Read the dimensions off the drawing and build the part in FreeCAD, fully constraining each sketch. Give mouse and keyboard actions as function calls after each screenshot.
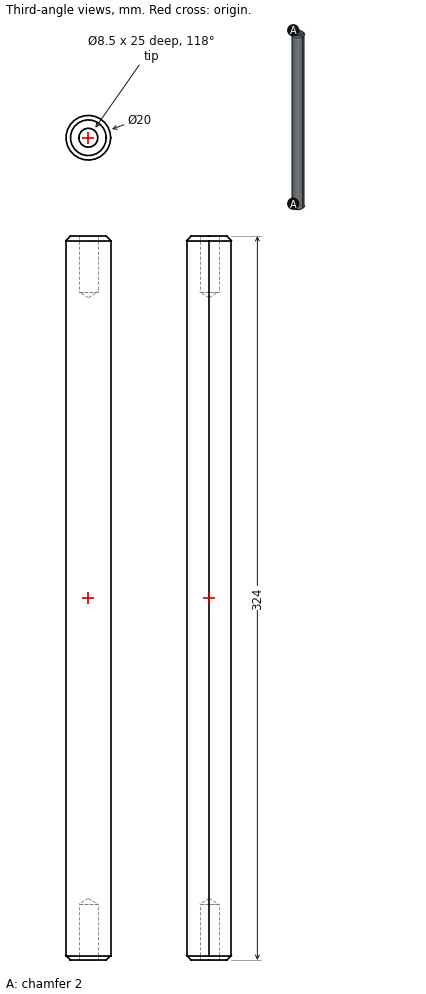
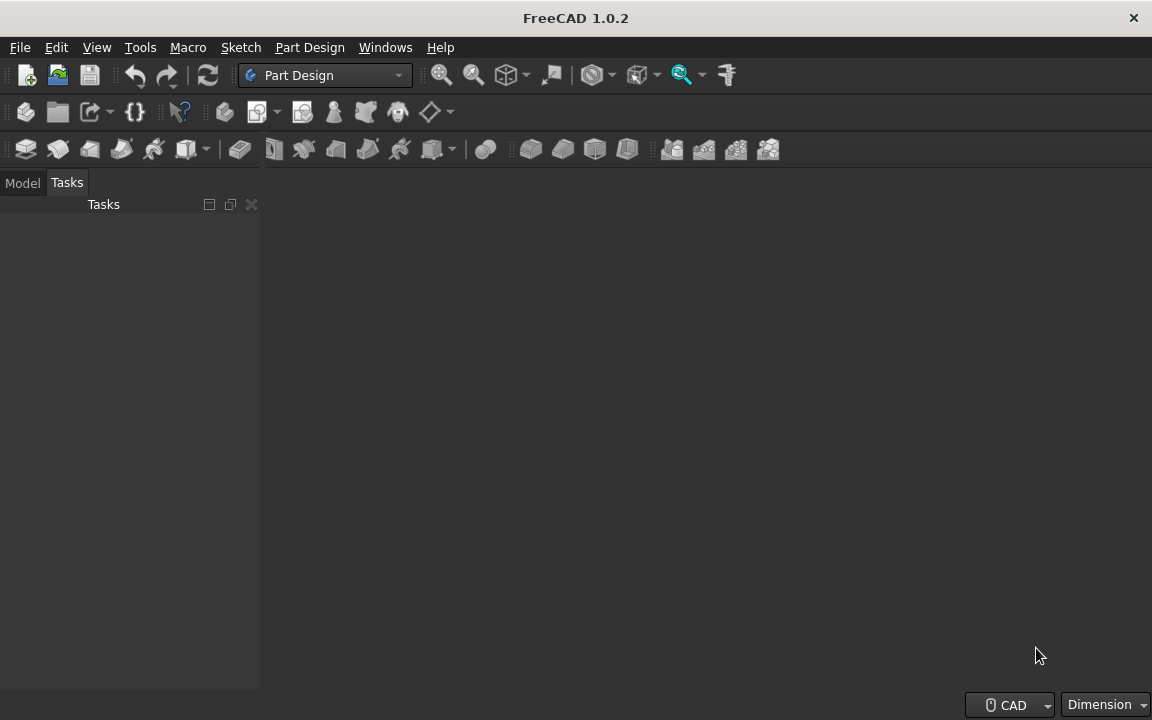
click(26, 76)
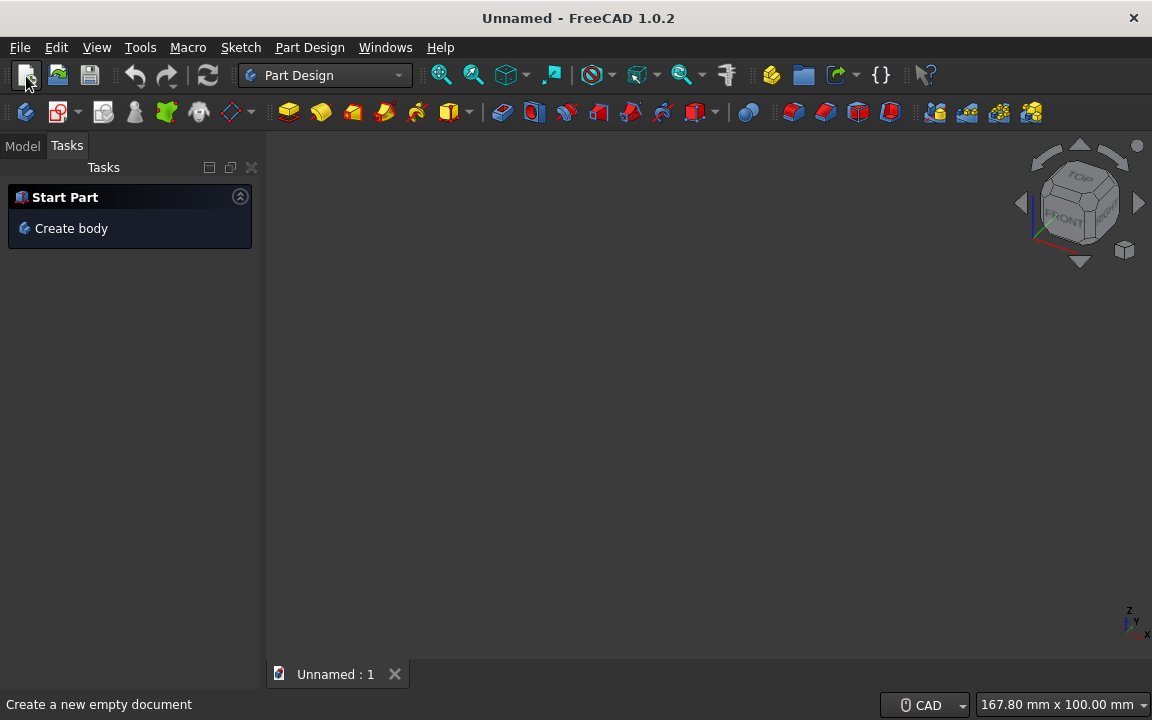
click(58, 112)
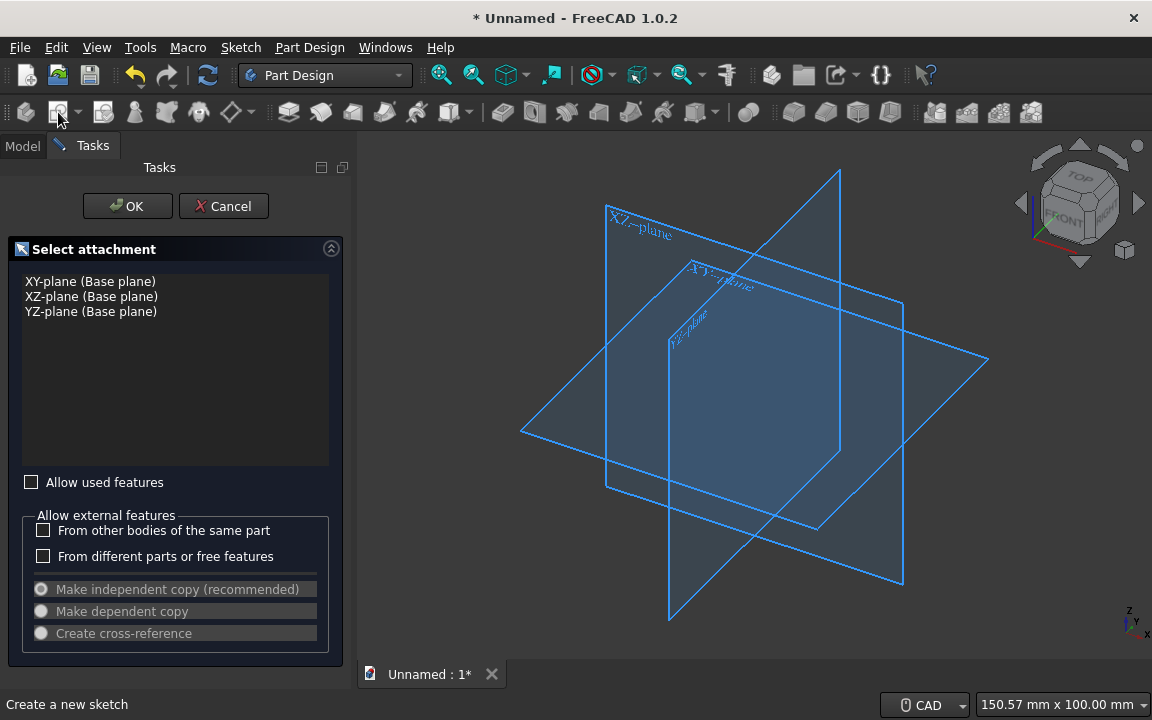
click(82, 282)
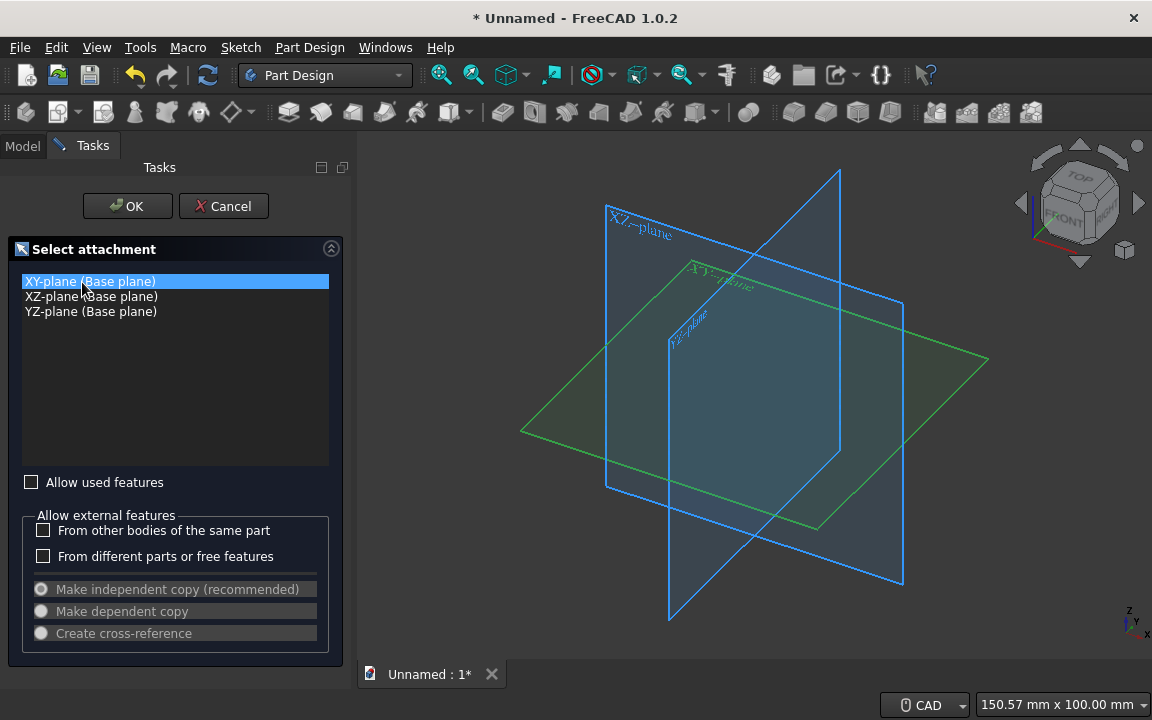
click(128, 206)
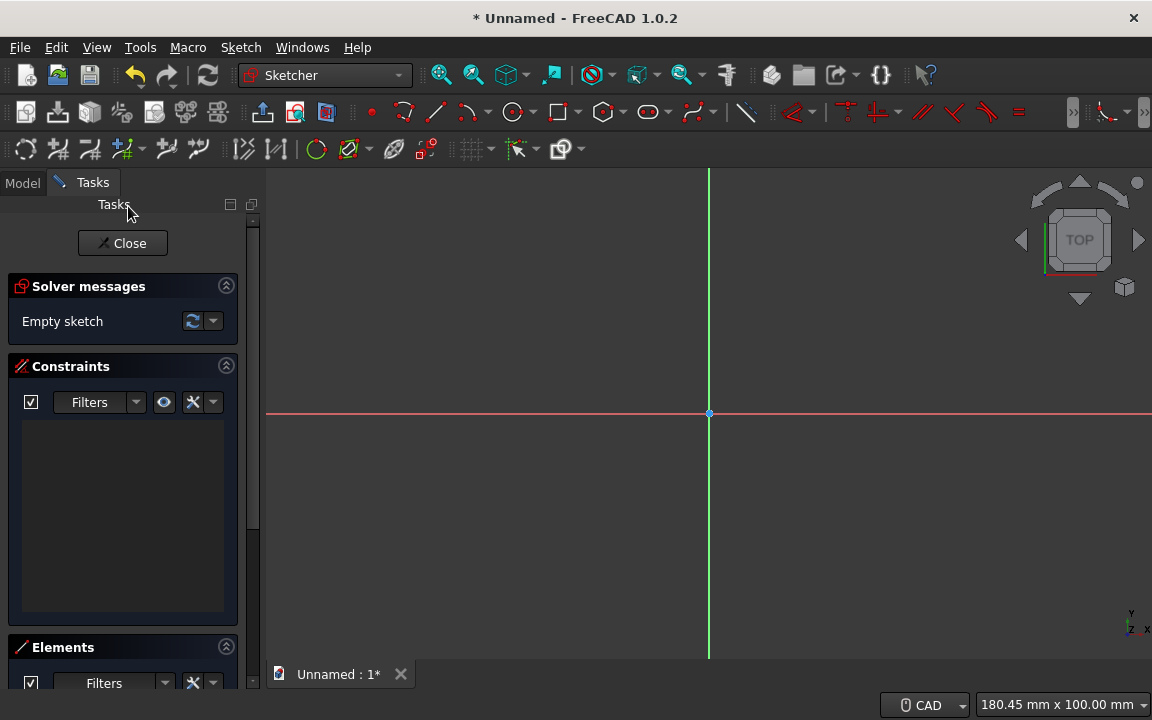
scroll(739, 414, up, 6)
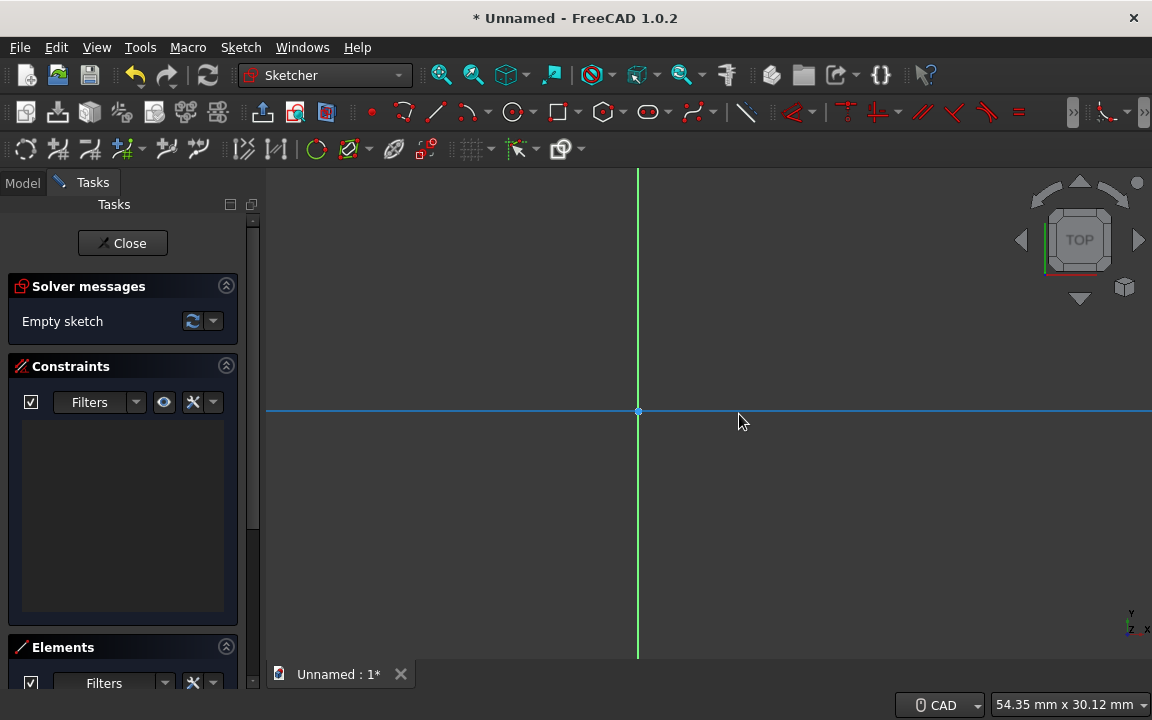
click(514, 112)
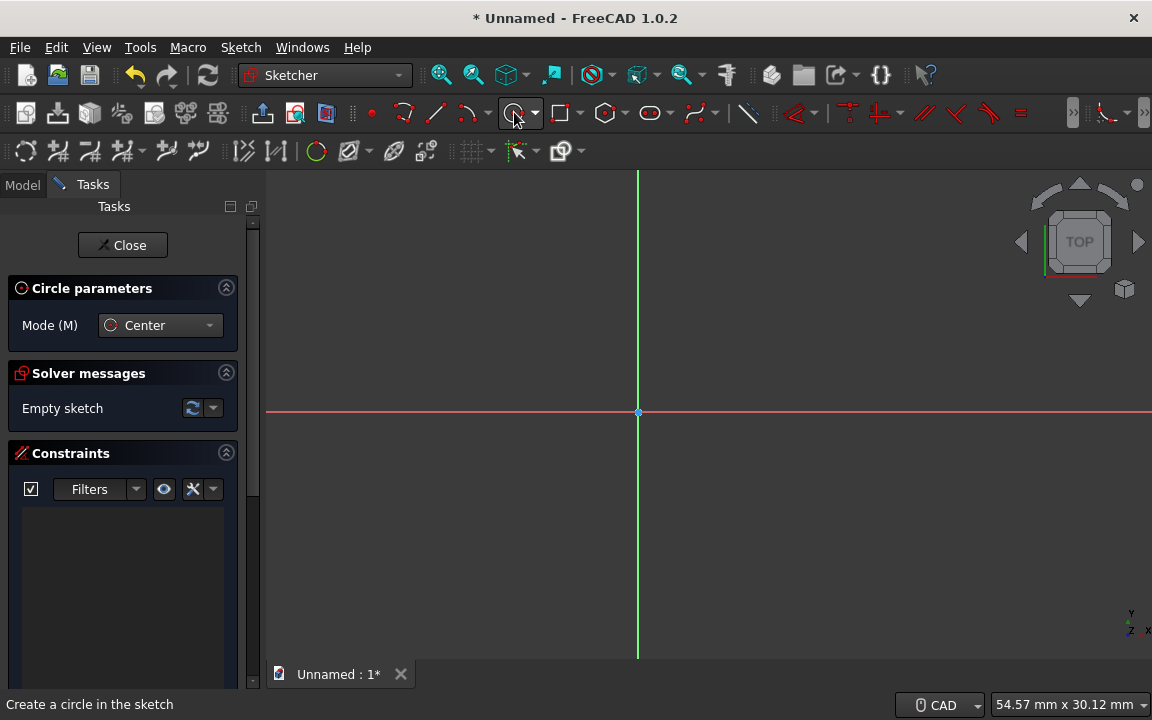
click(638, 412)
move(753, 297)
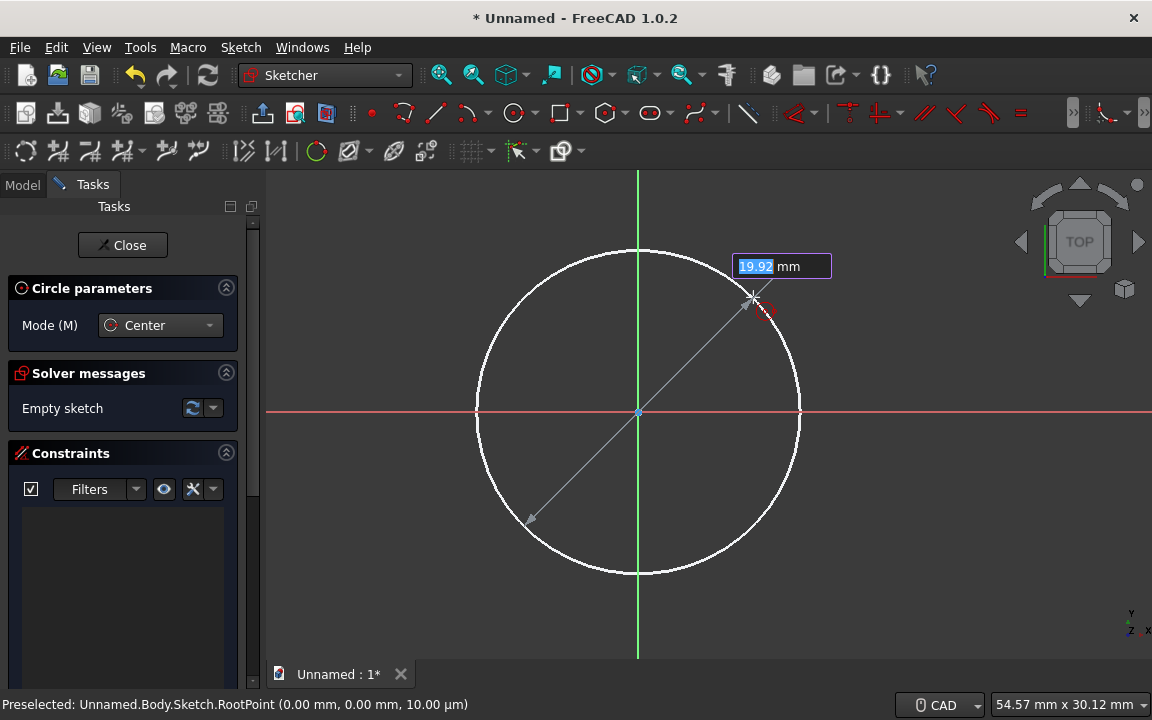
text(20)
key(Return)
key(Escape)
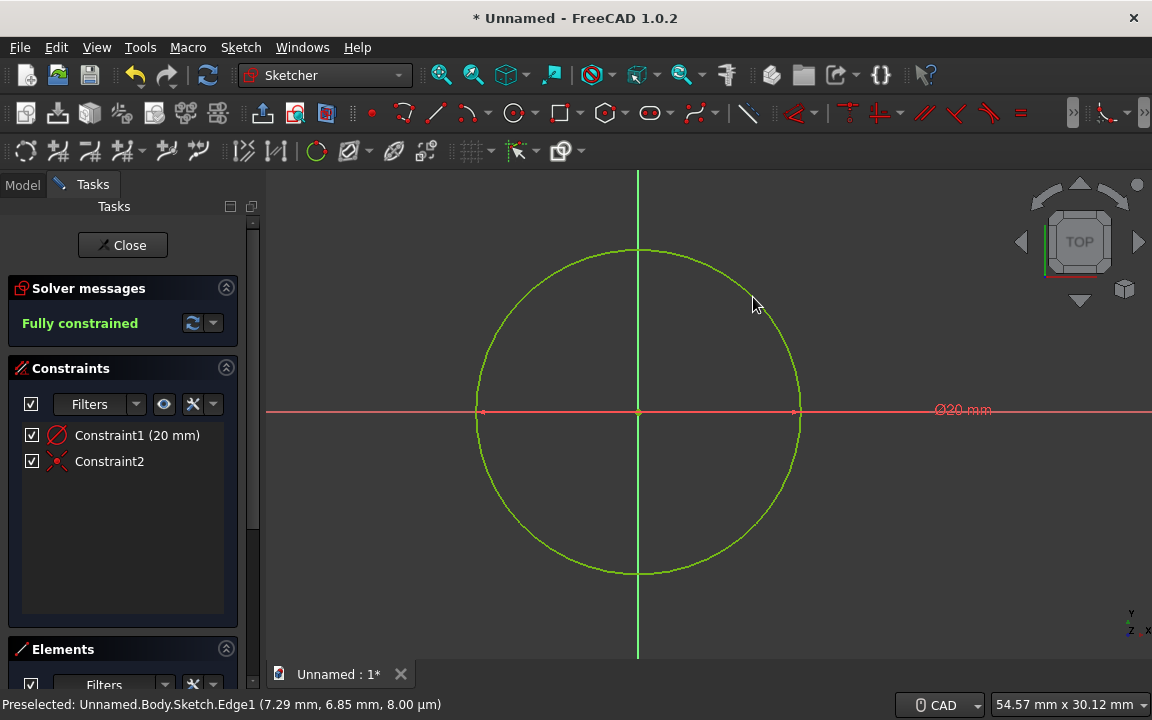
click(123, 245)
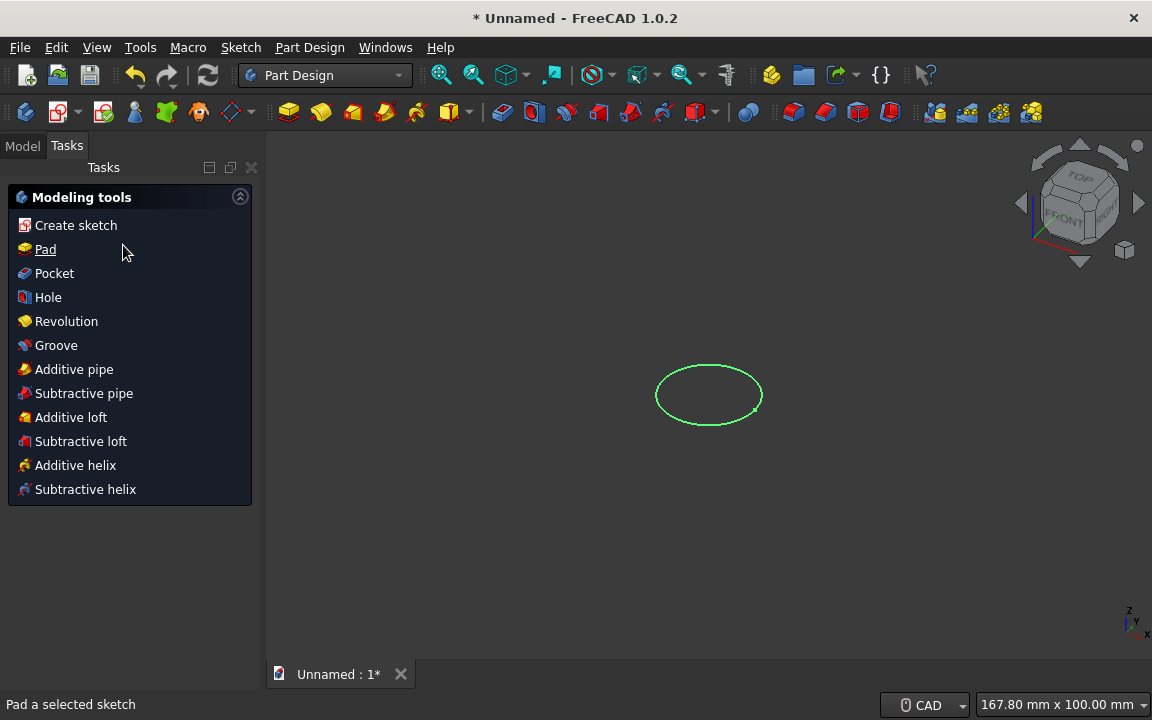
click(290, 112)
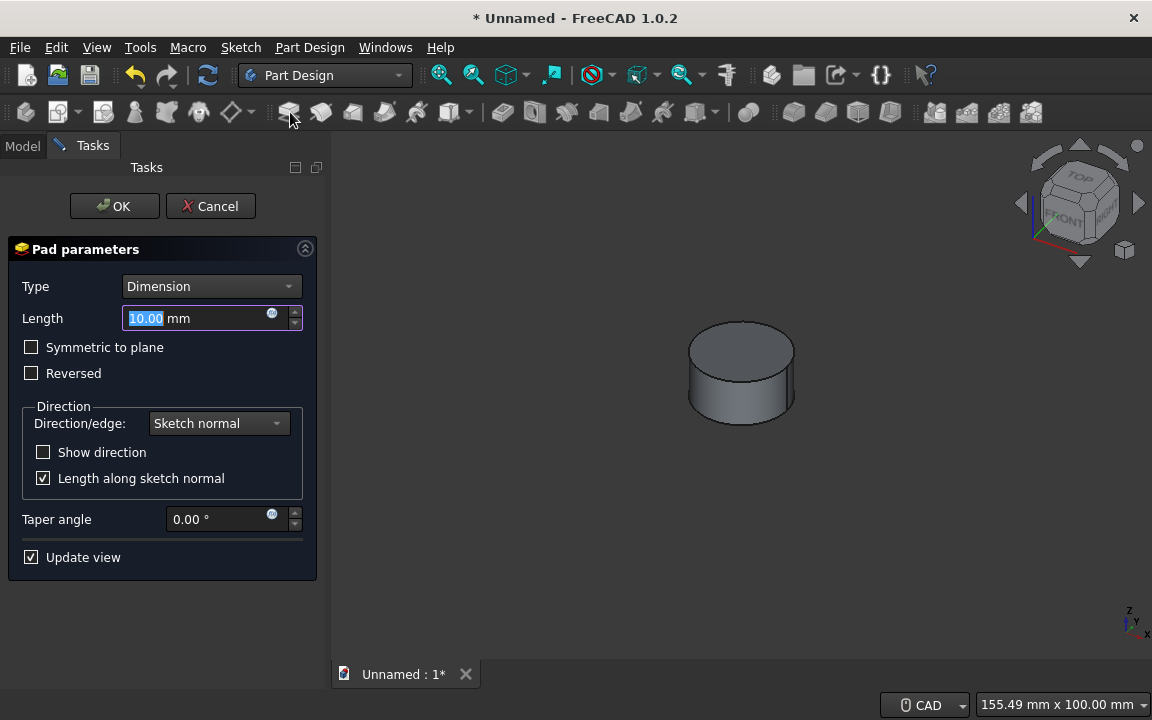
text(324)
key(Tab)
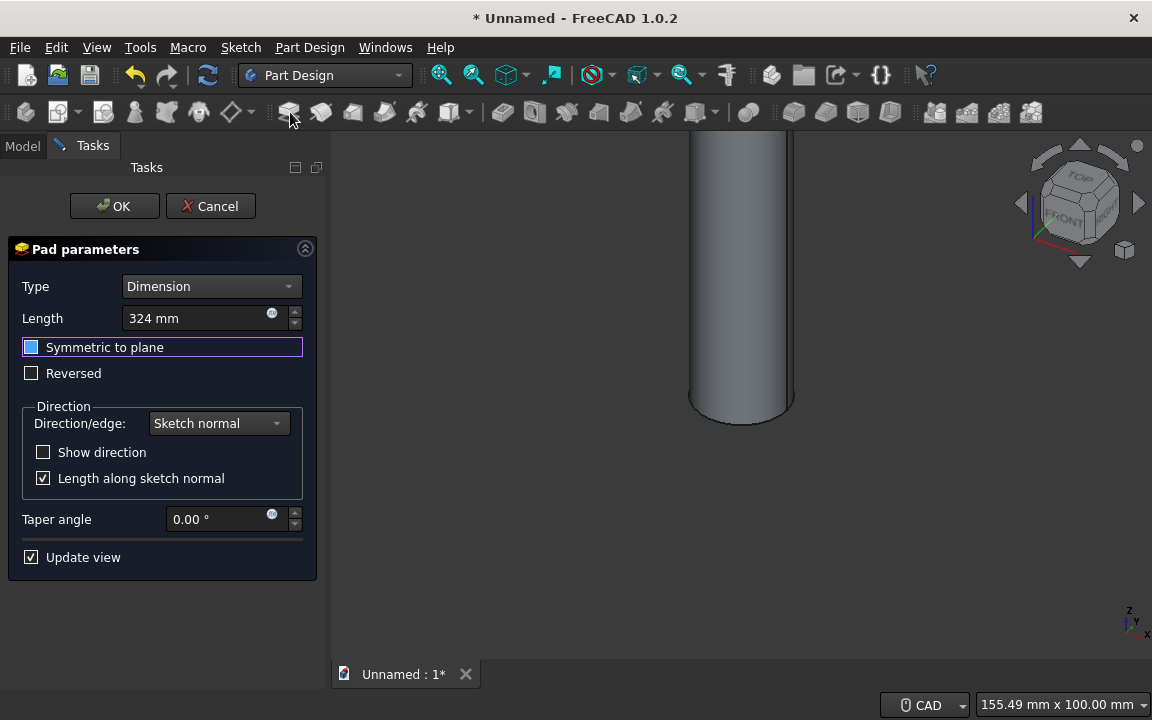
click(30, 347)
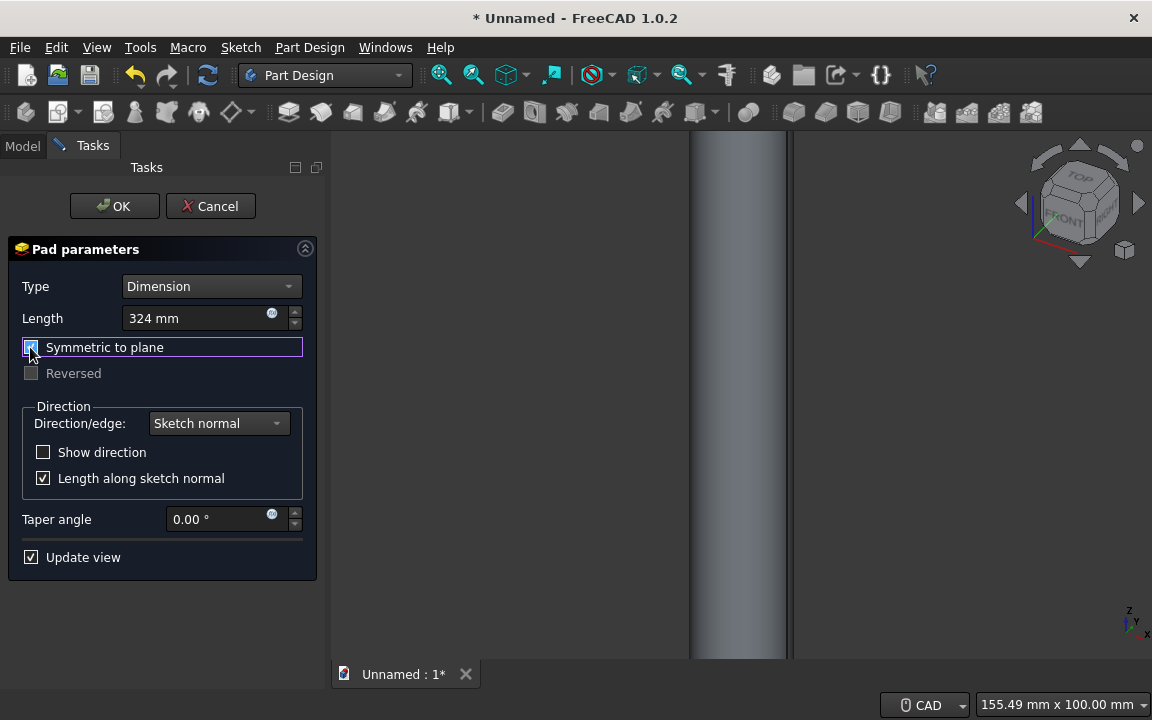
click(115, 206)